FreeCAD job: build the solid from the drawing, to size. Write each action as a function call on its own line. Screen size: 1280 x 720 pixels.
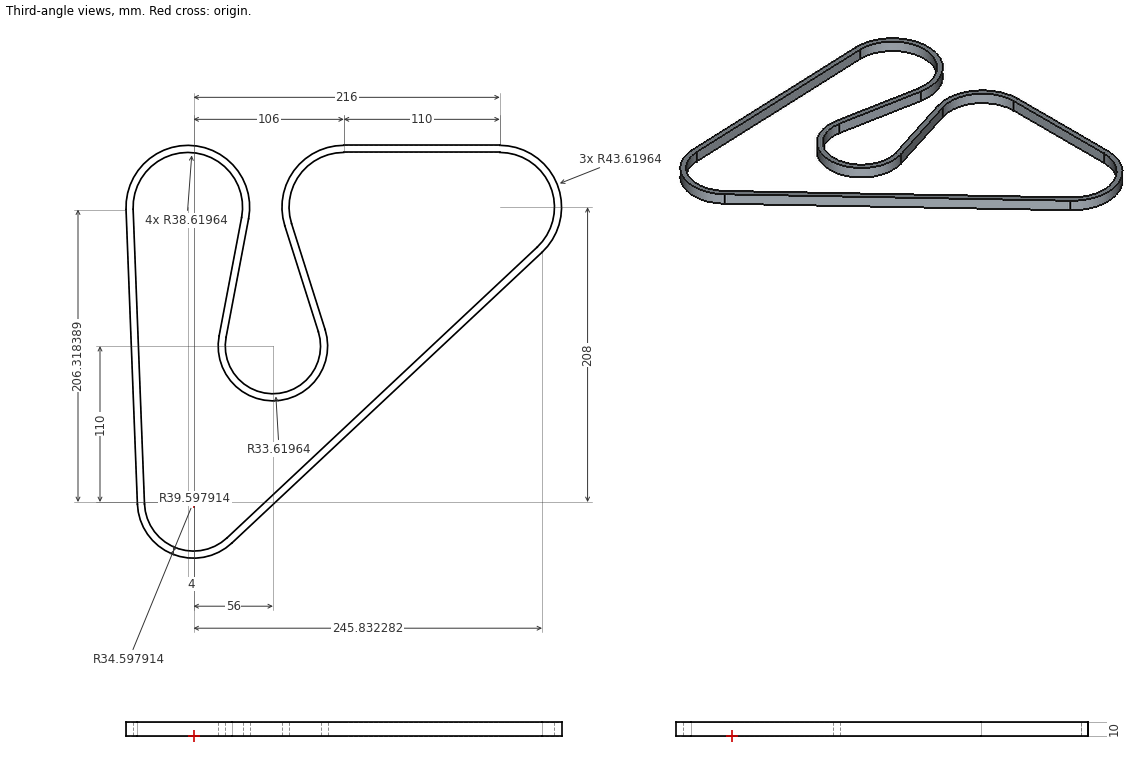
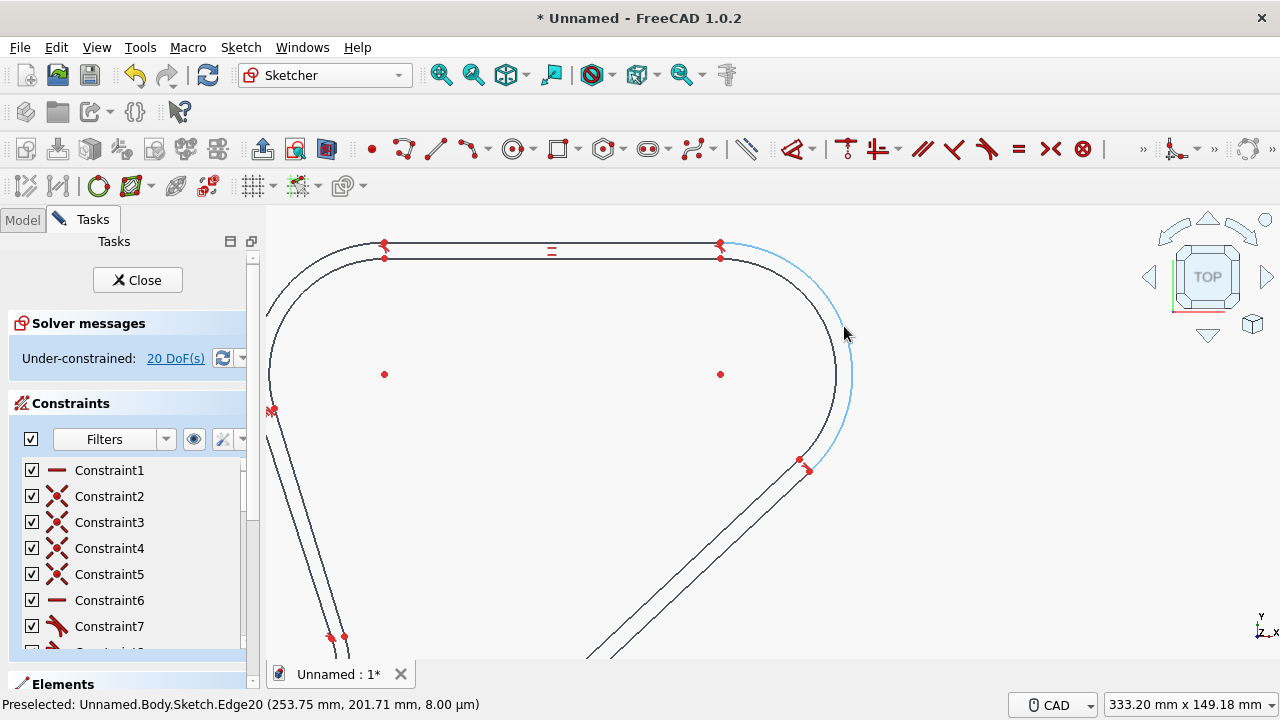
click(843, 327)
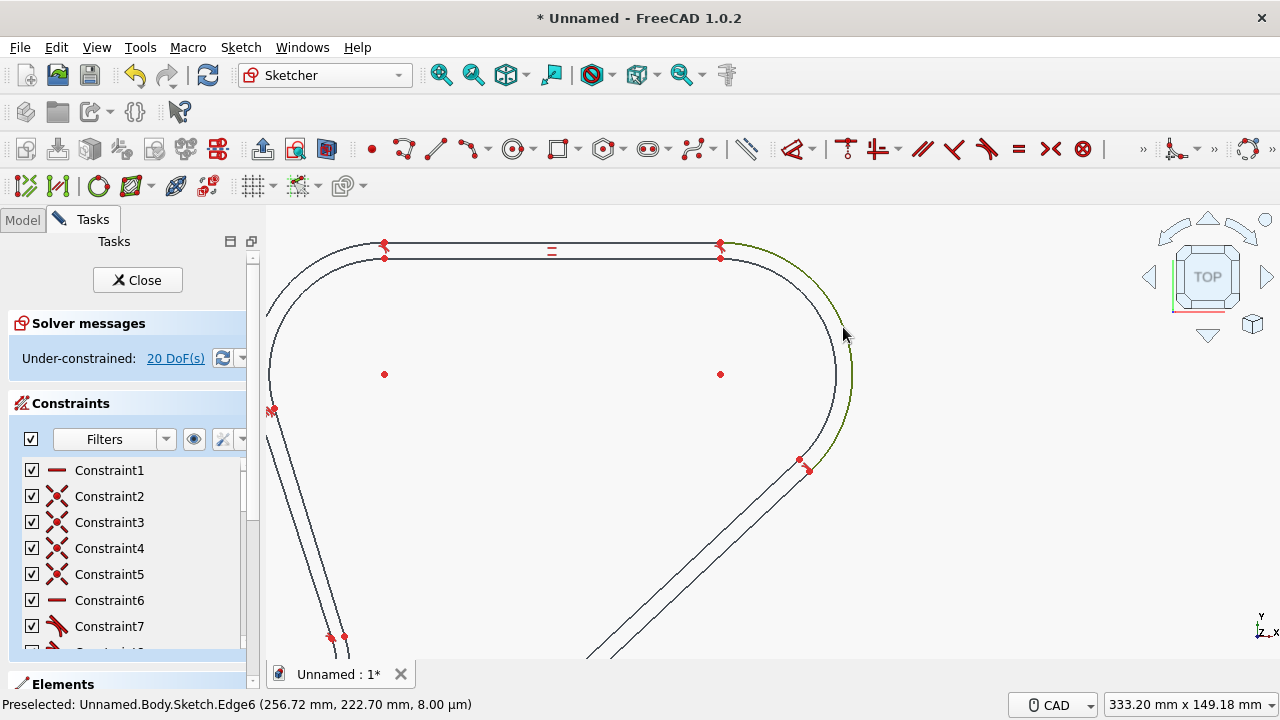
click(314, 263)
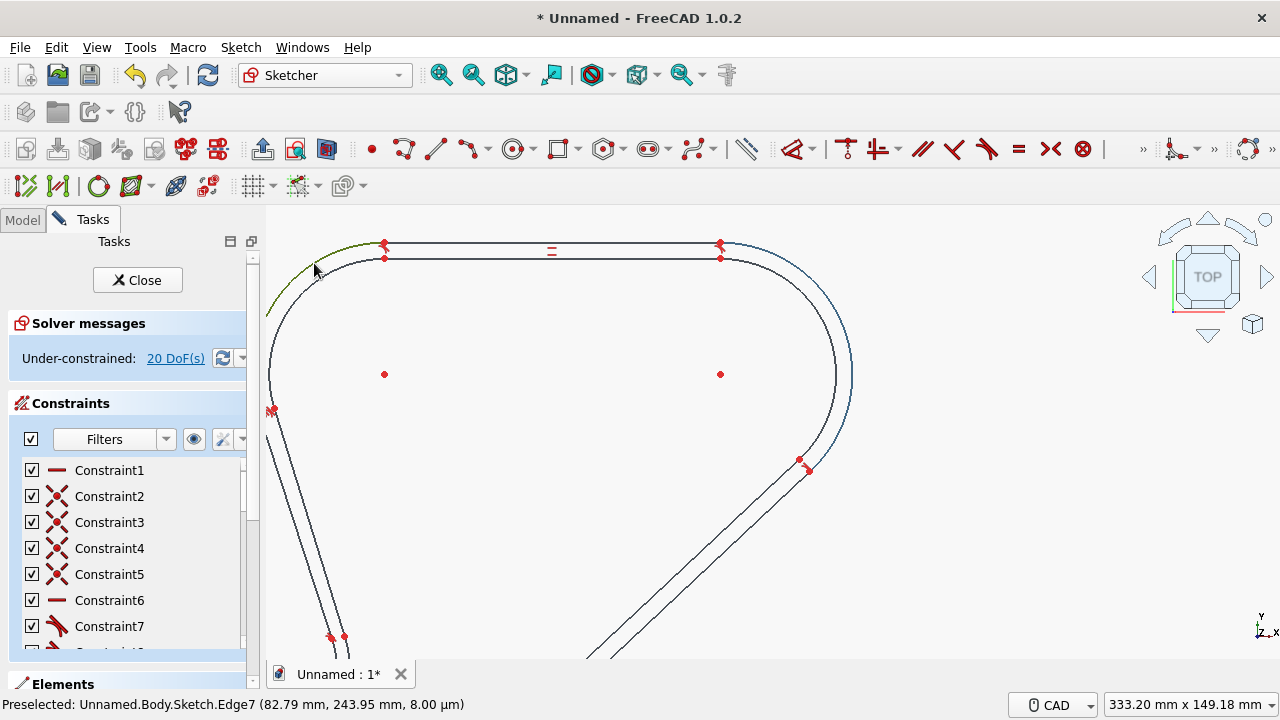
scroll(844, 326, down, 6)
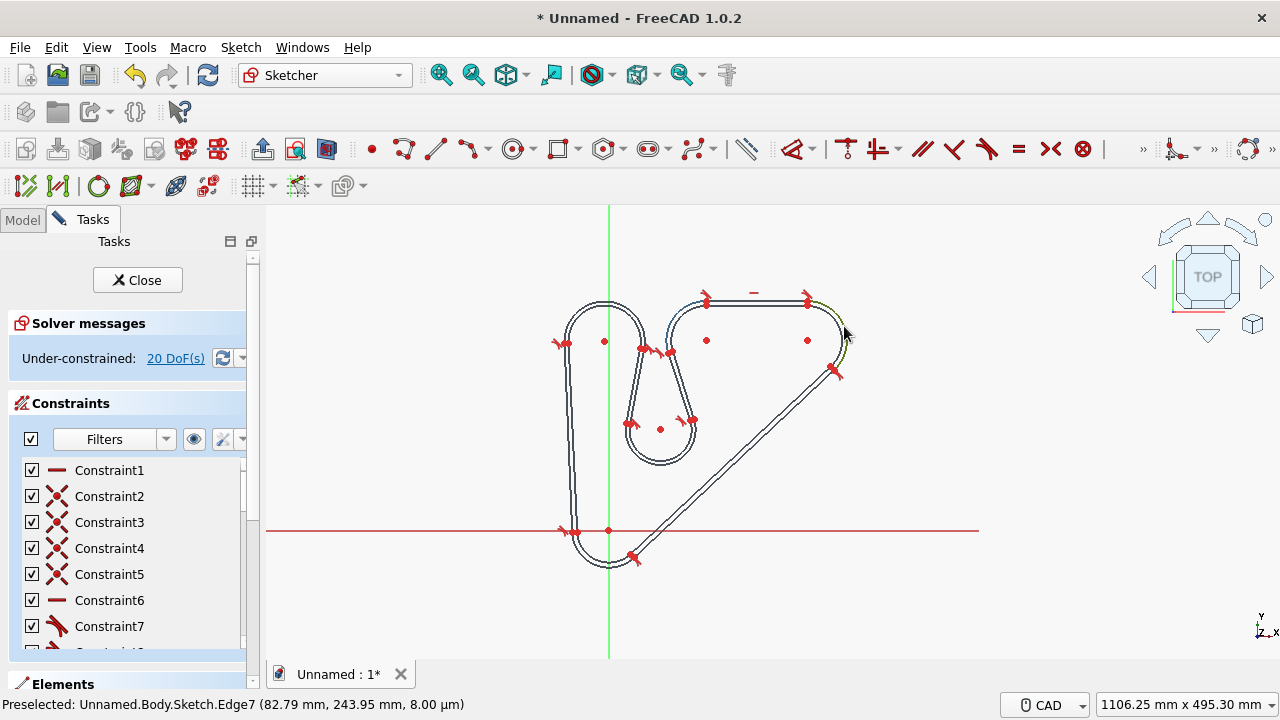
scroll(632, 312, up, 7)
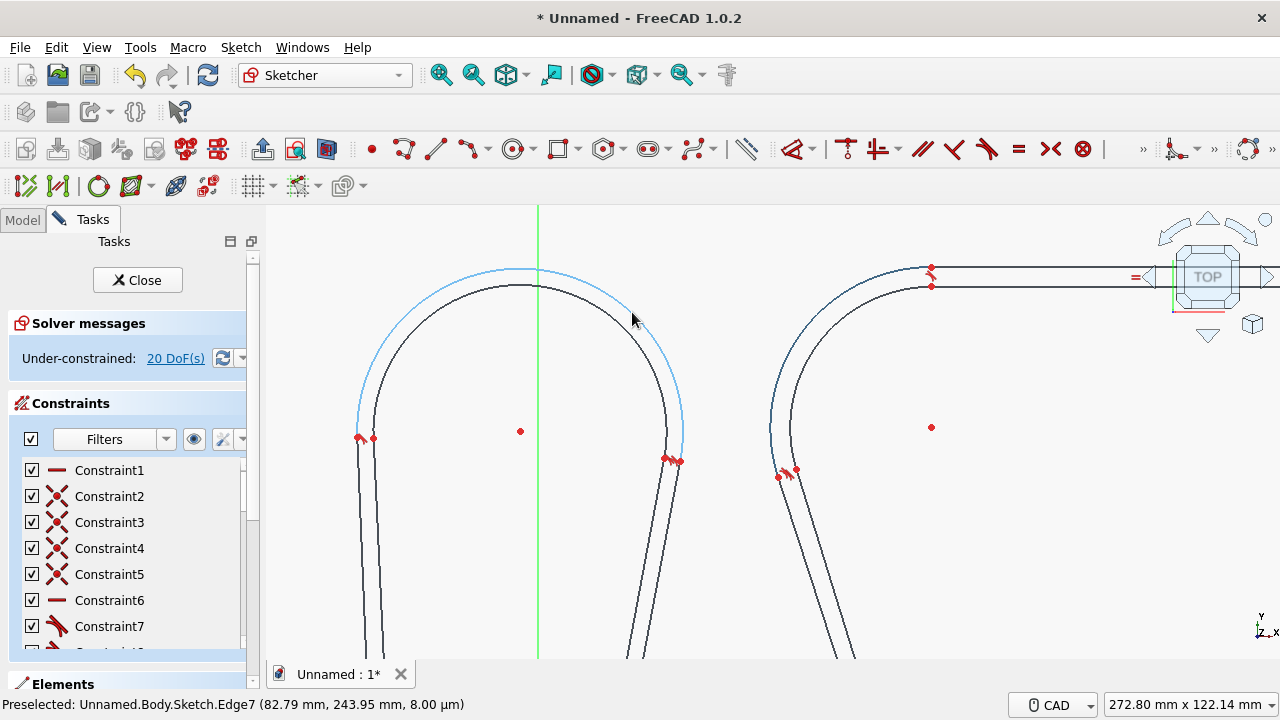
click(631, 312)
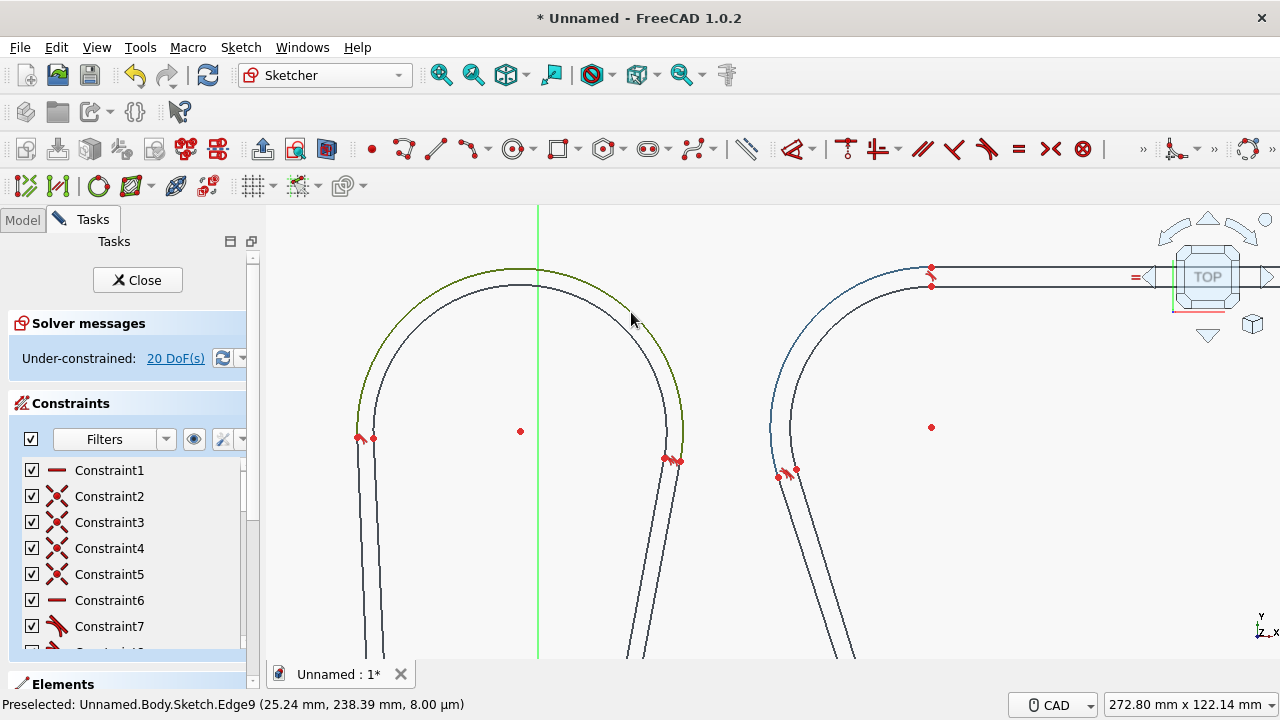
click(1020, 150)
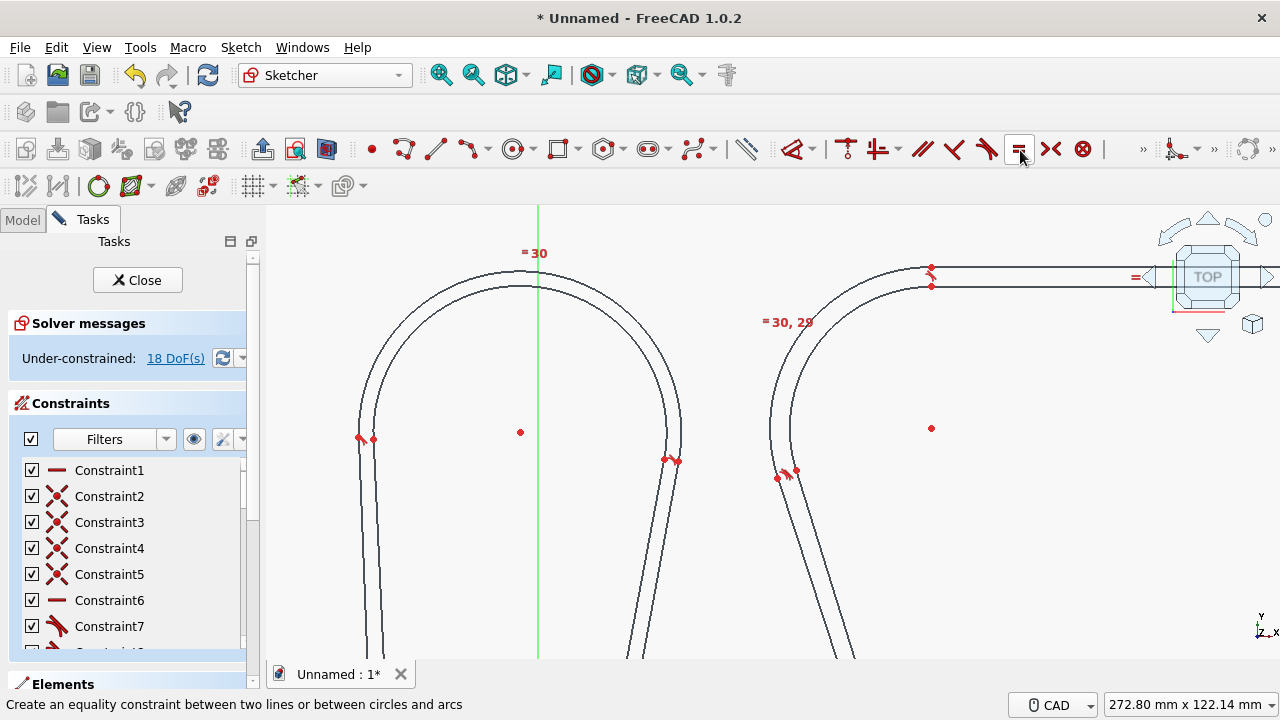
click(619, 325)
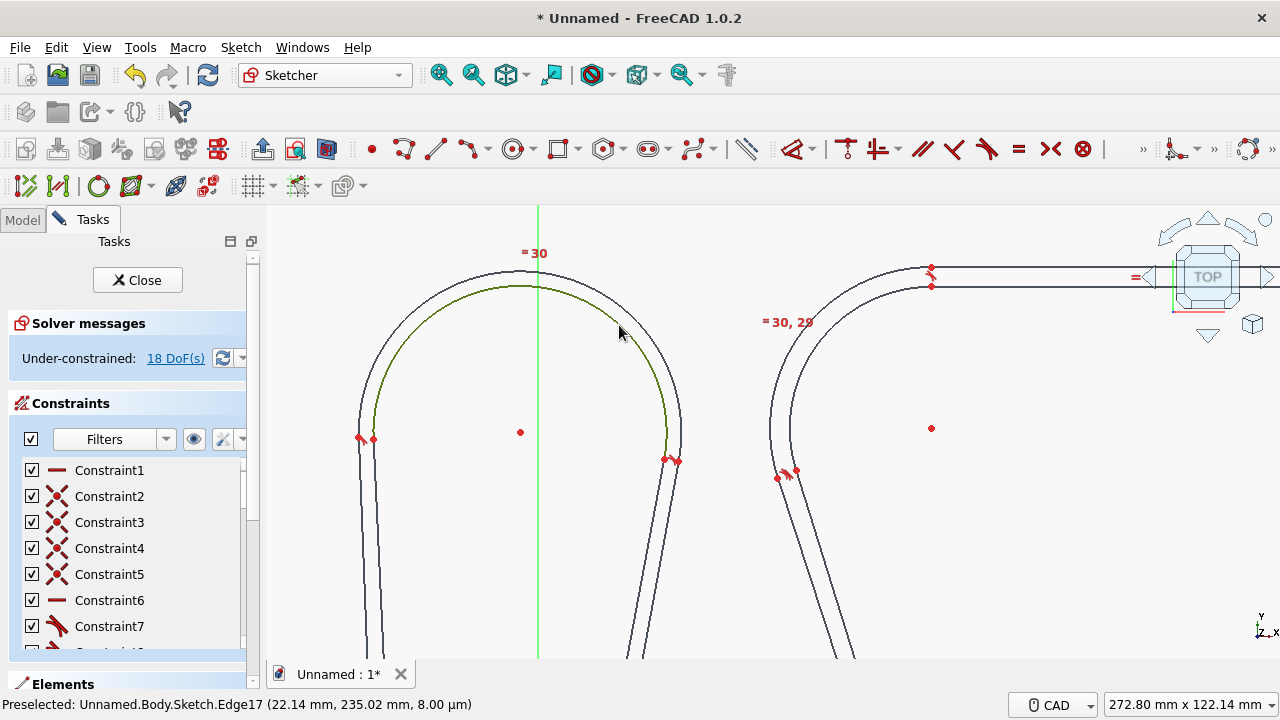
scroll(632, 312, down, 7)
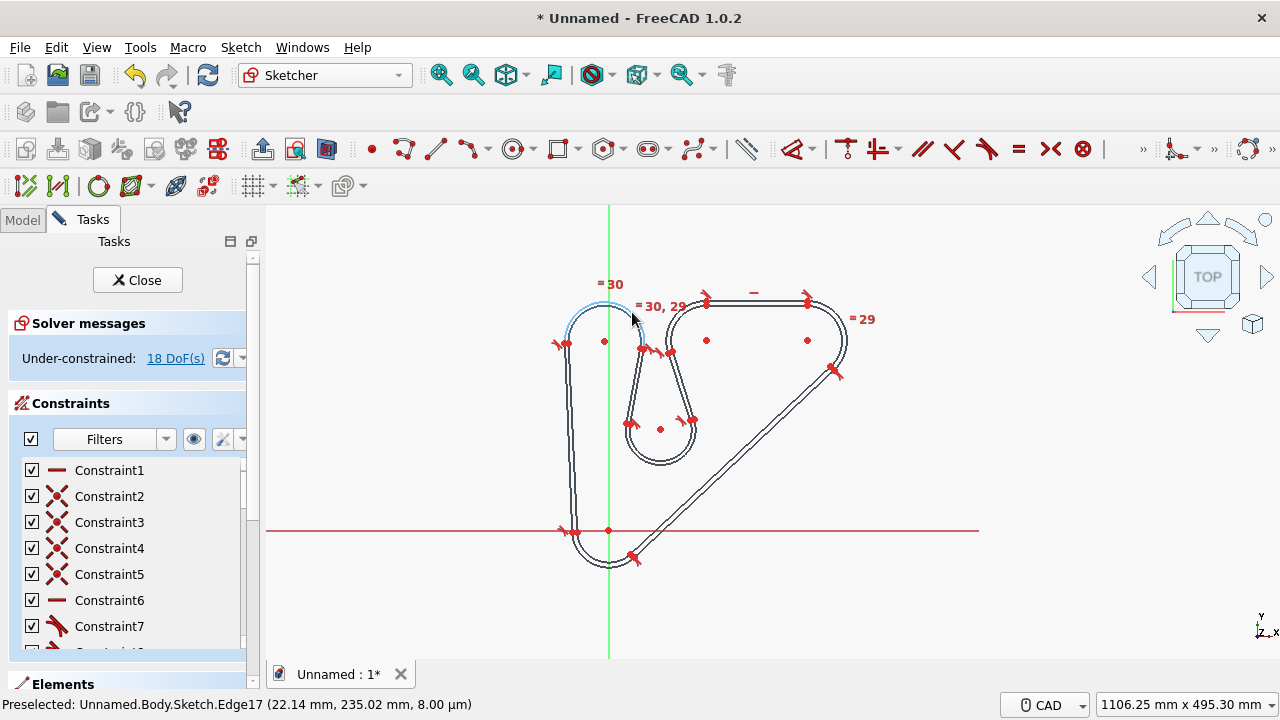
scroll(639, 457, up, 7)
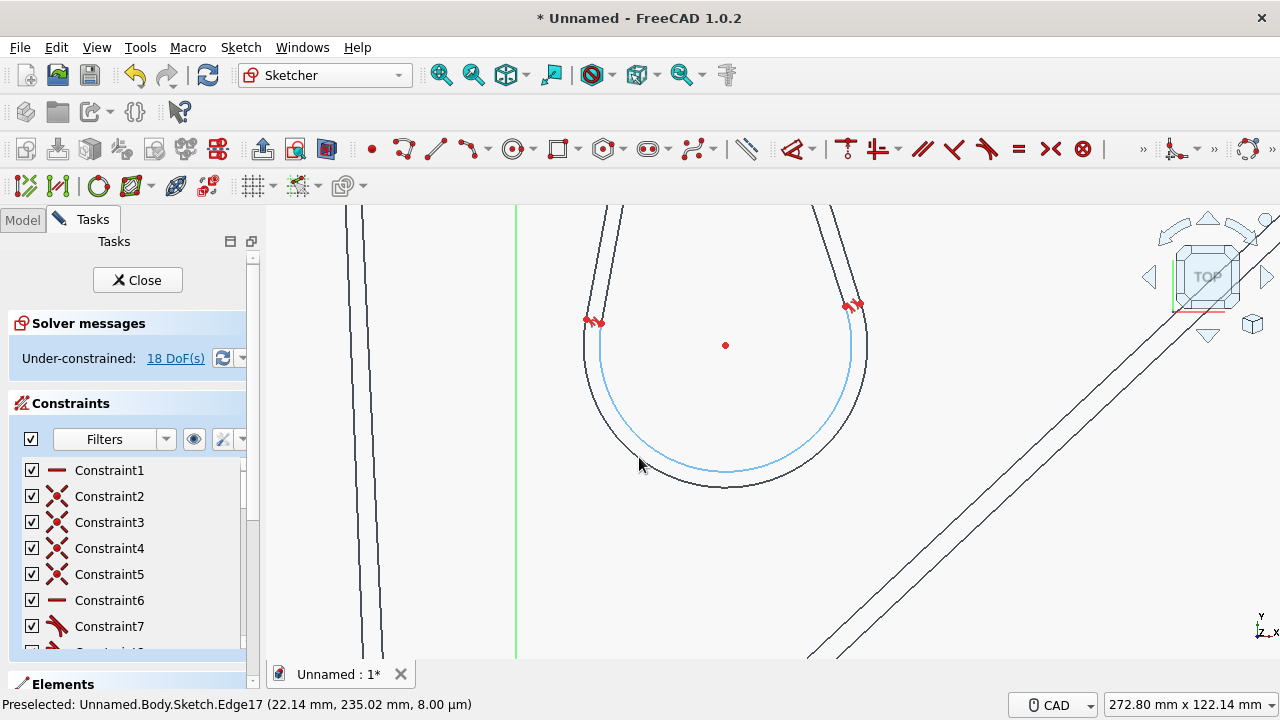
click(638, 457)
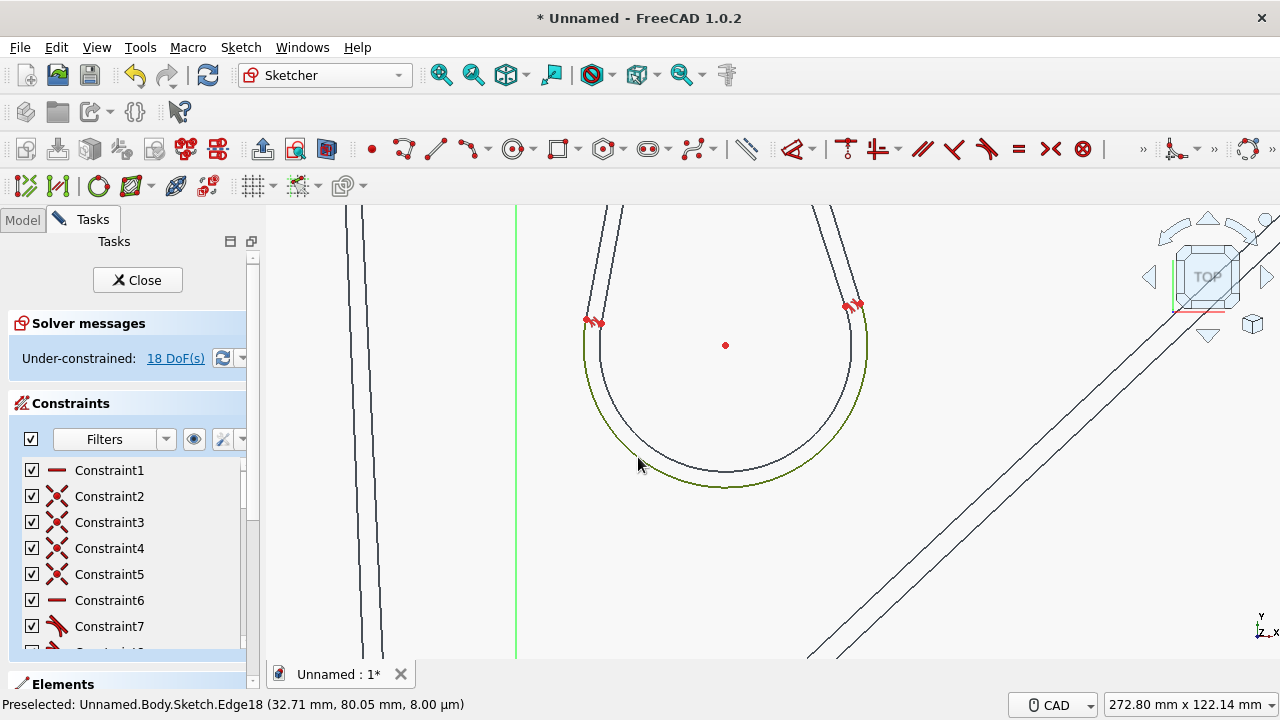
scroll(639, 457, down, 7)